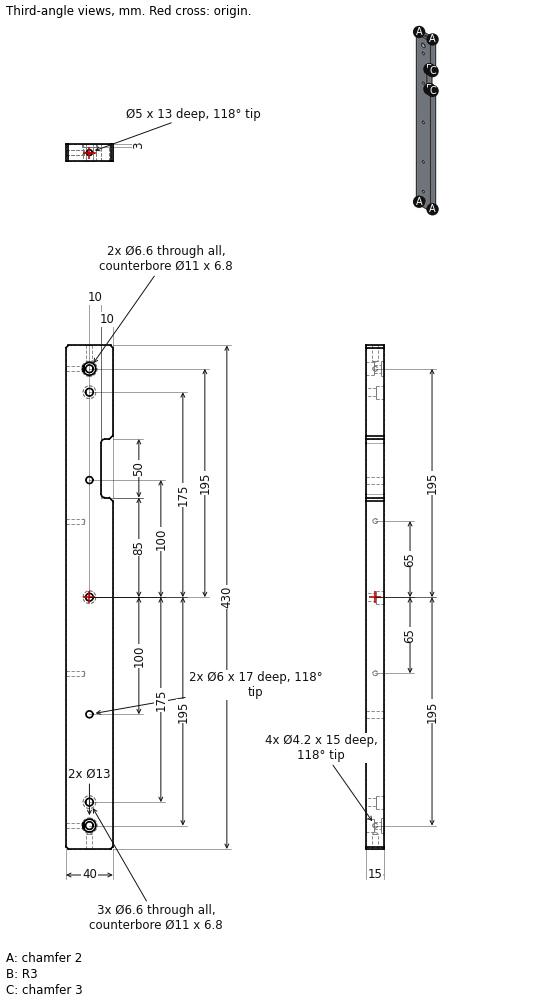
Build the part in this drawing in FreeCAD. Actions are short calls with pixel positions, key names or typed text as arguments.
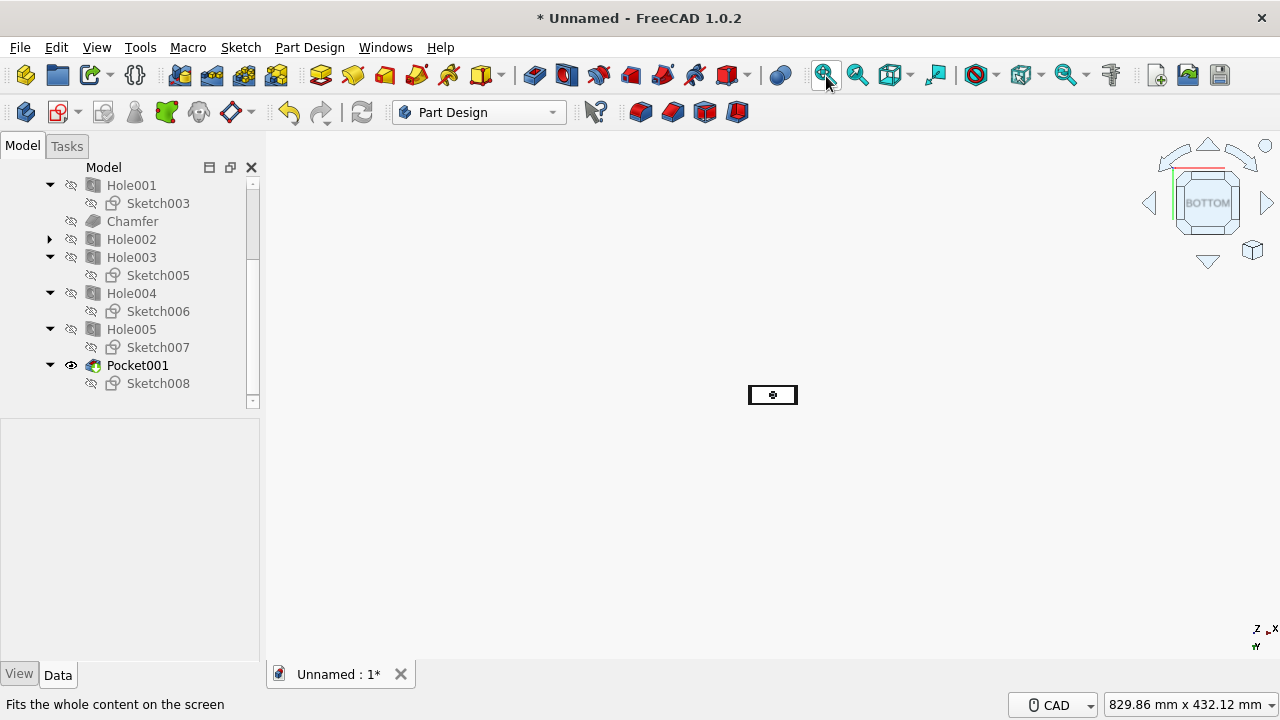
click(826, 76)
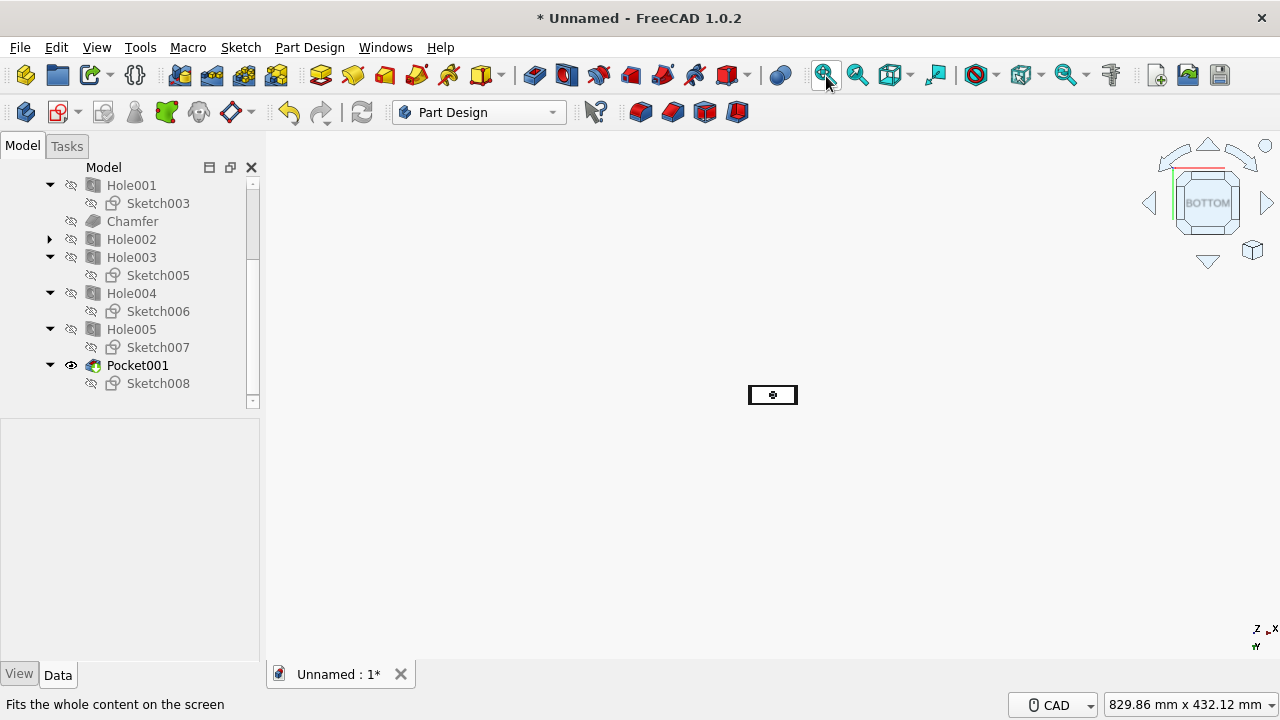
scroll(785, 394, up, 4)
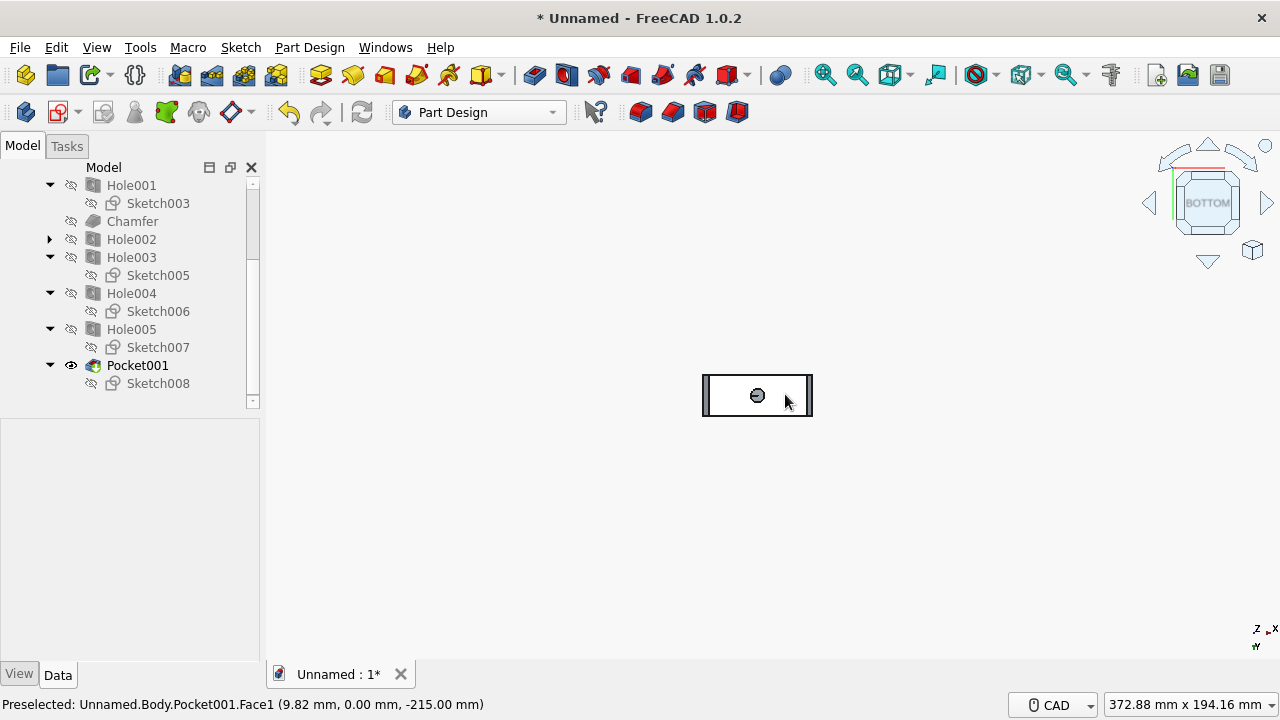
click(826, 76)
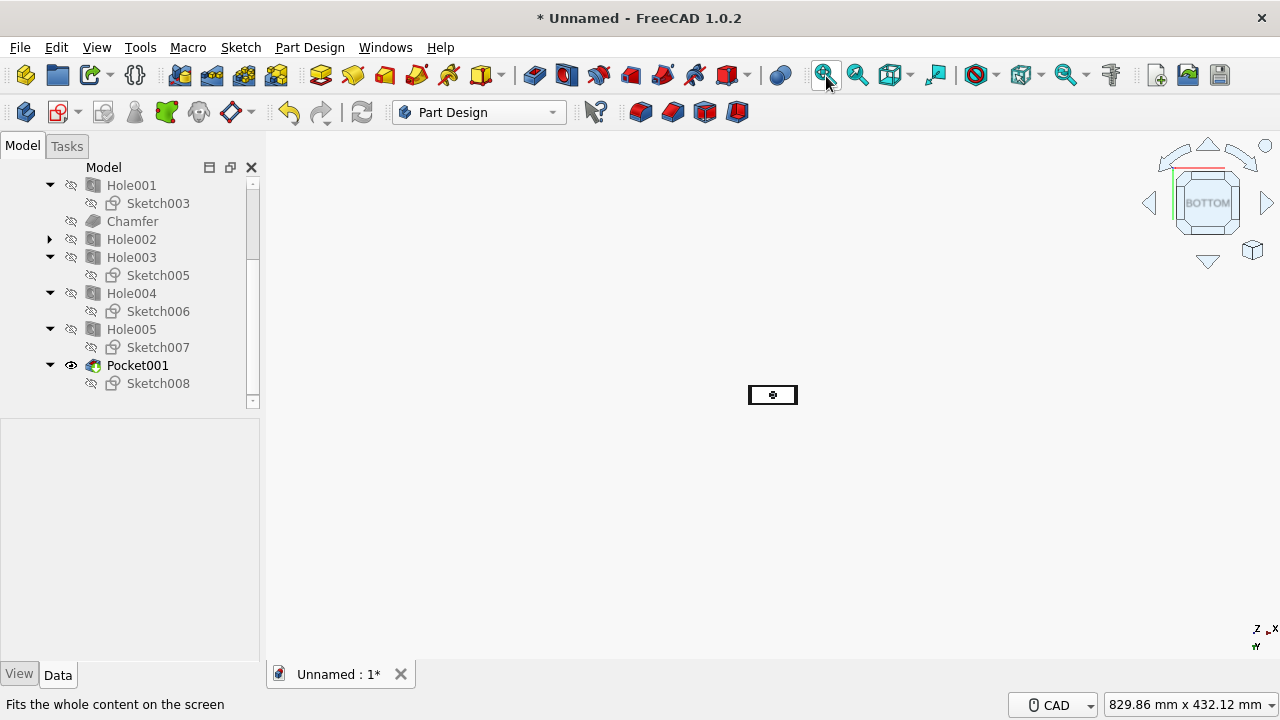
key(4)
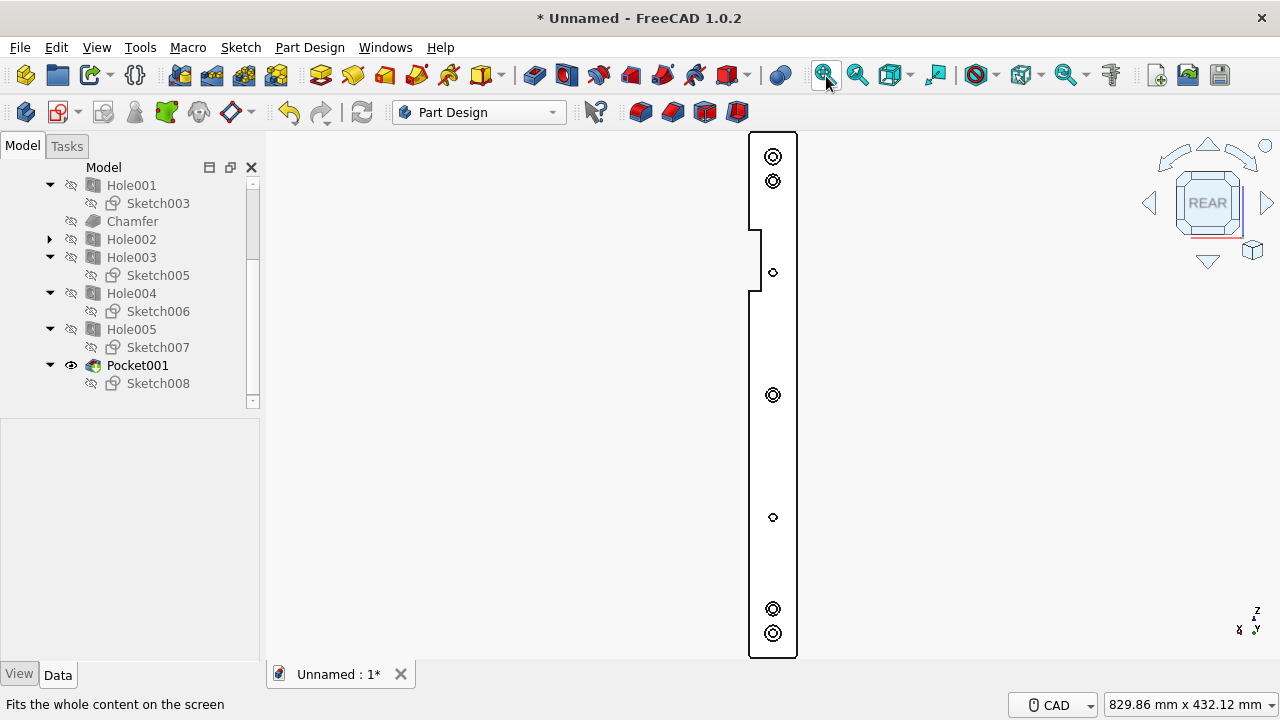
scroll(761, 290, up, 4)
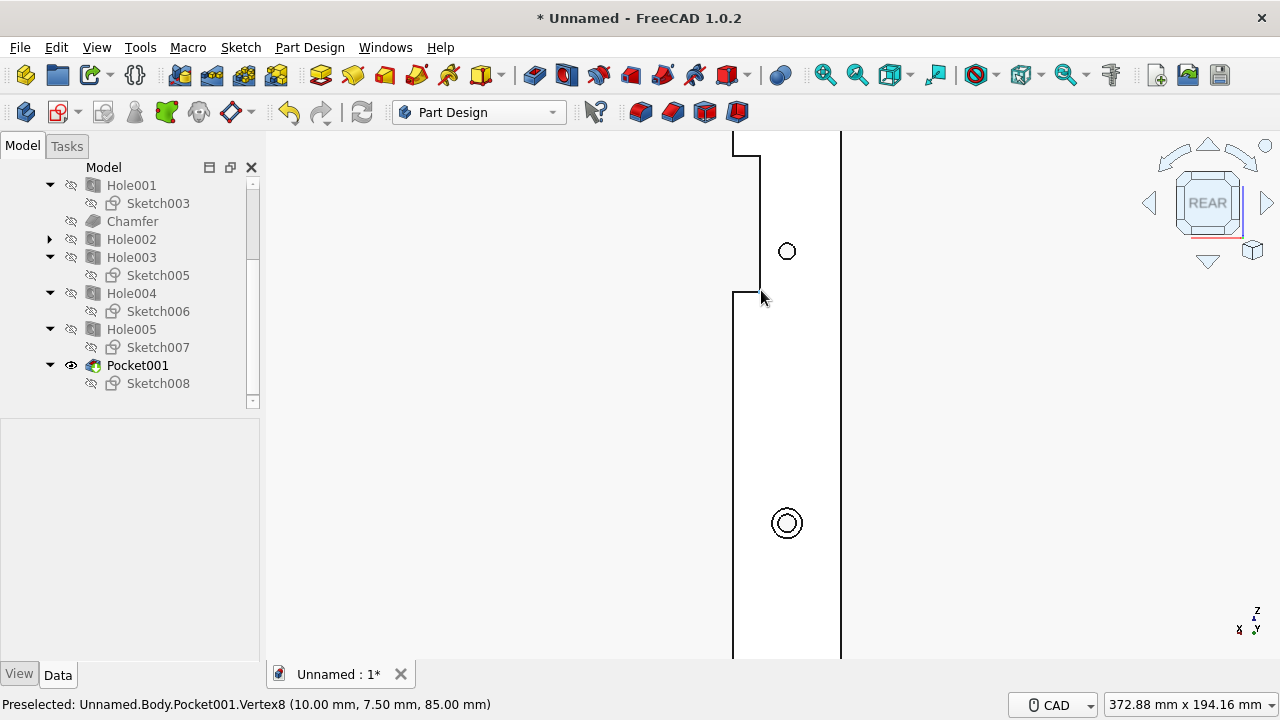
click(826, 76)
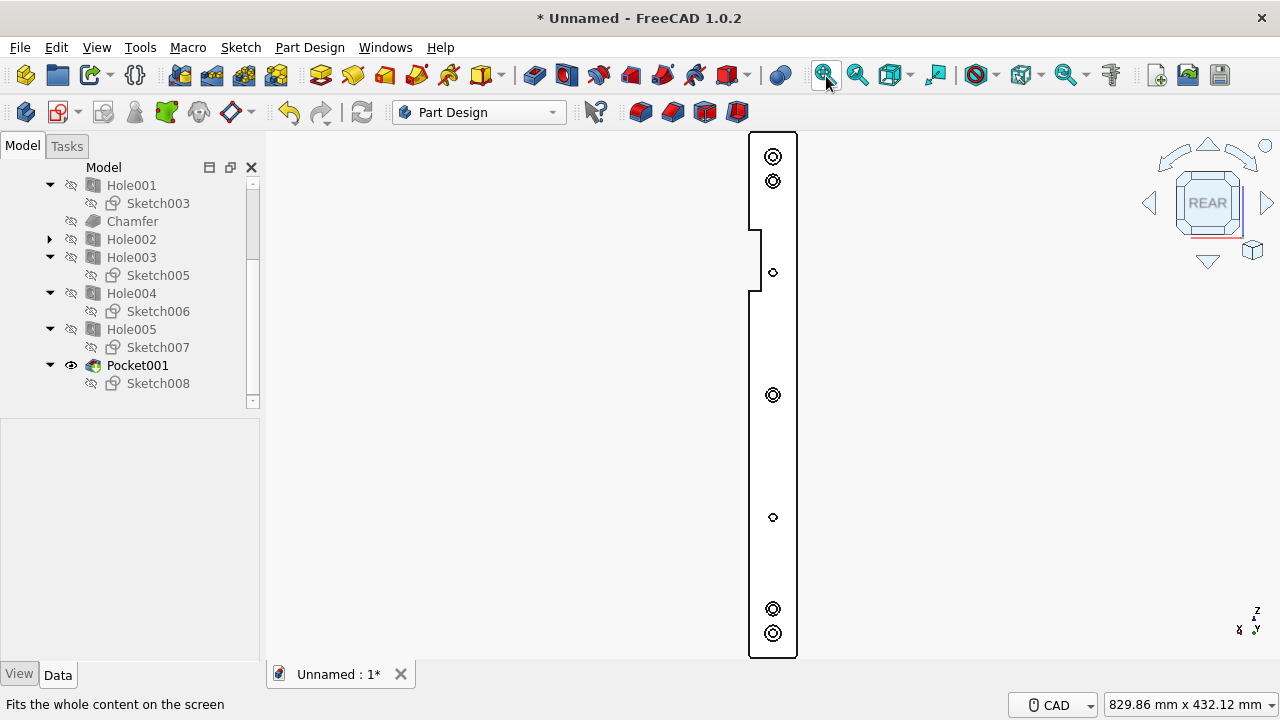
key(6)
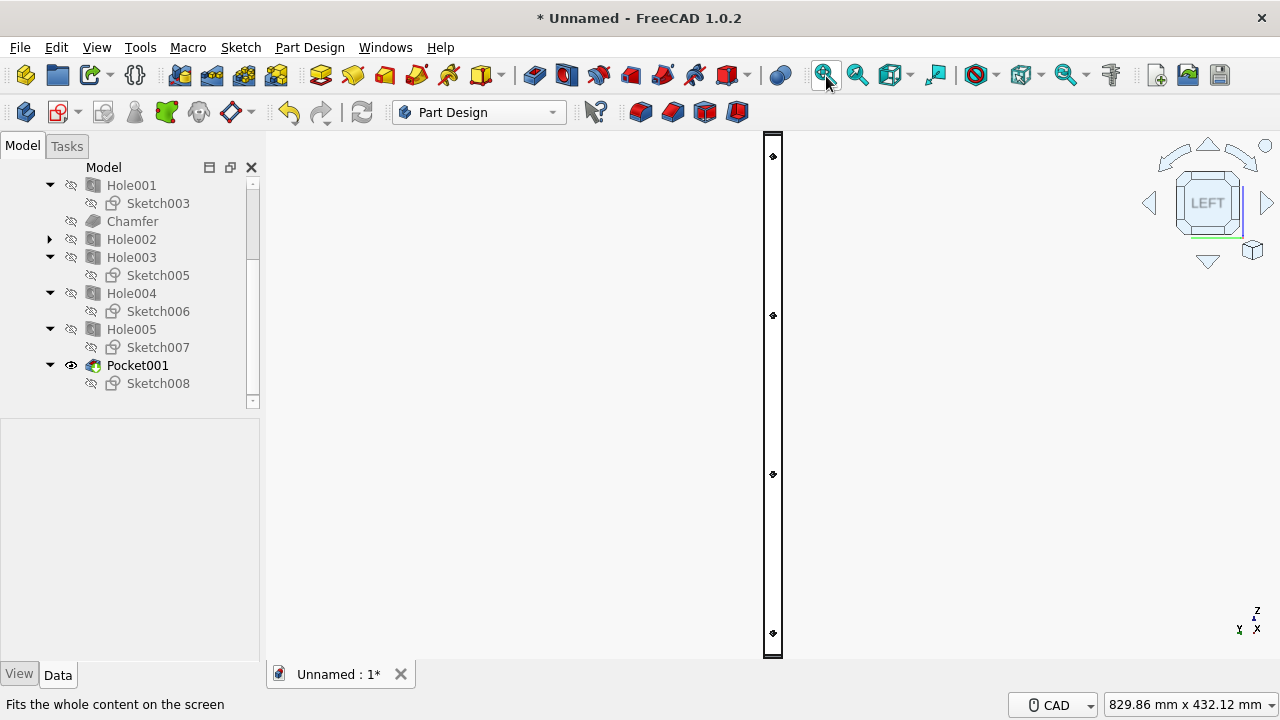
scroll(773, 290, up, 4)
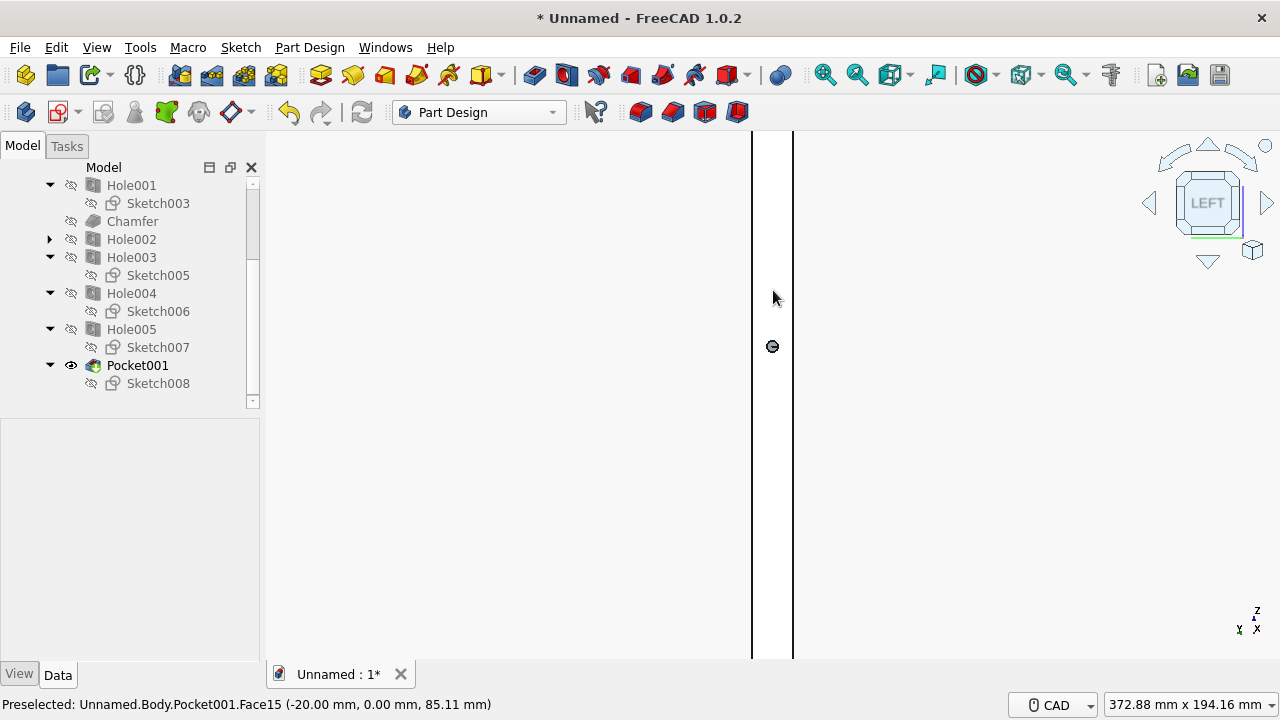
click(826, 76)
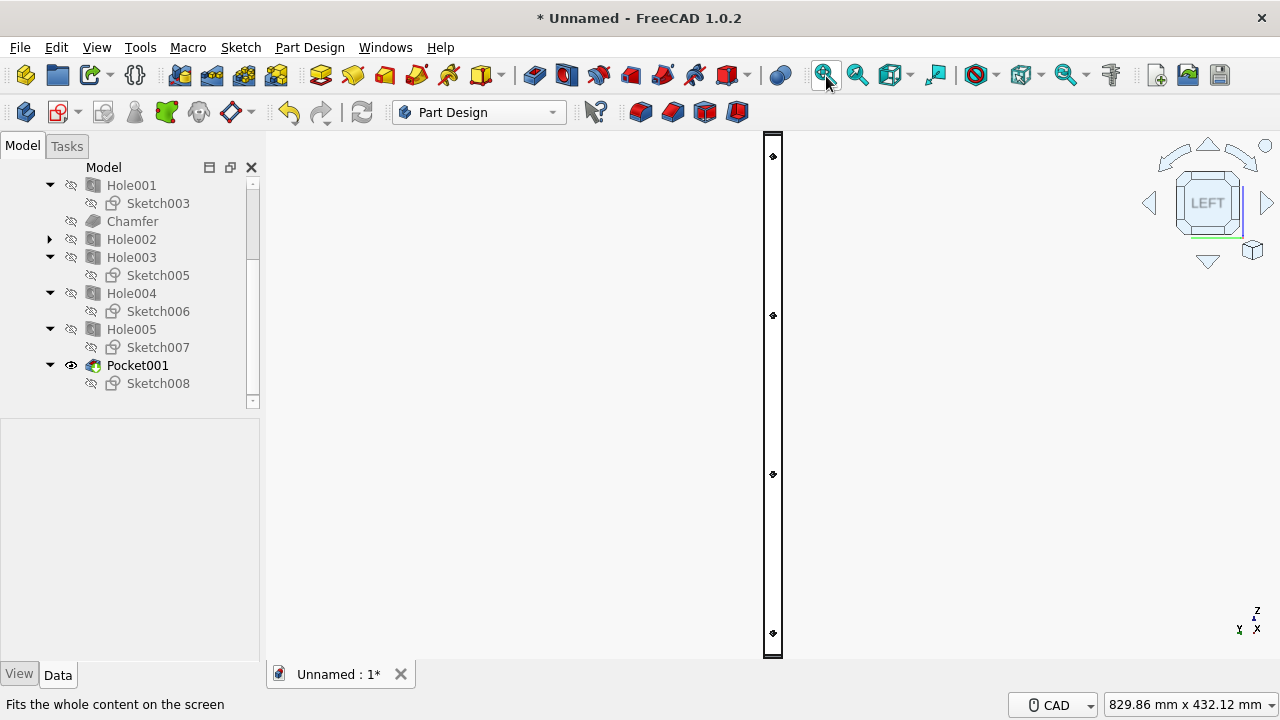
key(v)
key(3)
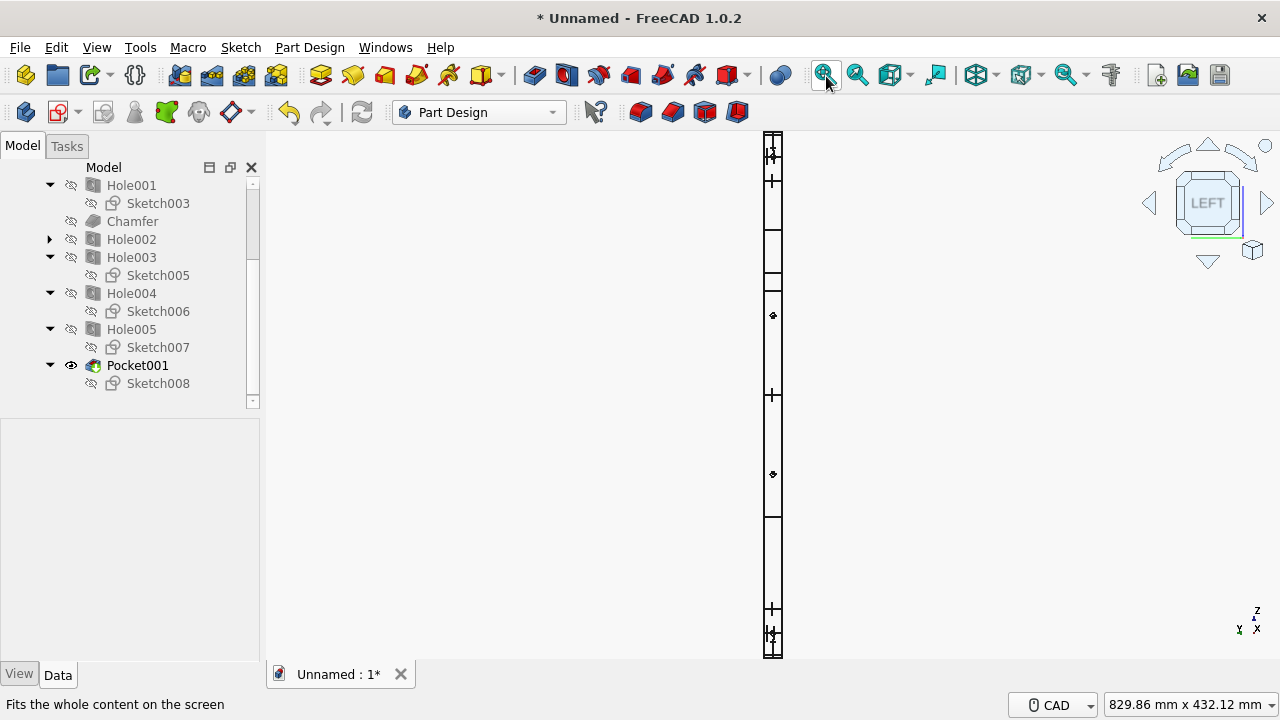
key(0)